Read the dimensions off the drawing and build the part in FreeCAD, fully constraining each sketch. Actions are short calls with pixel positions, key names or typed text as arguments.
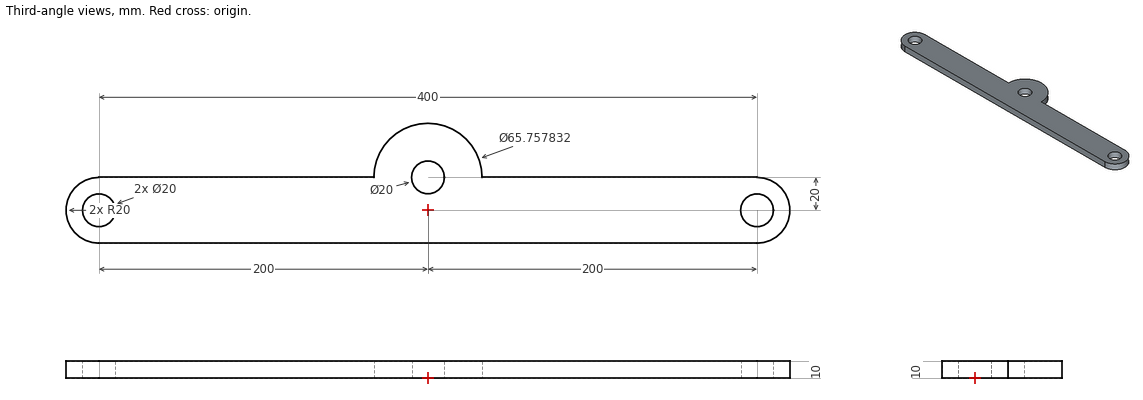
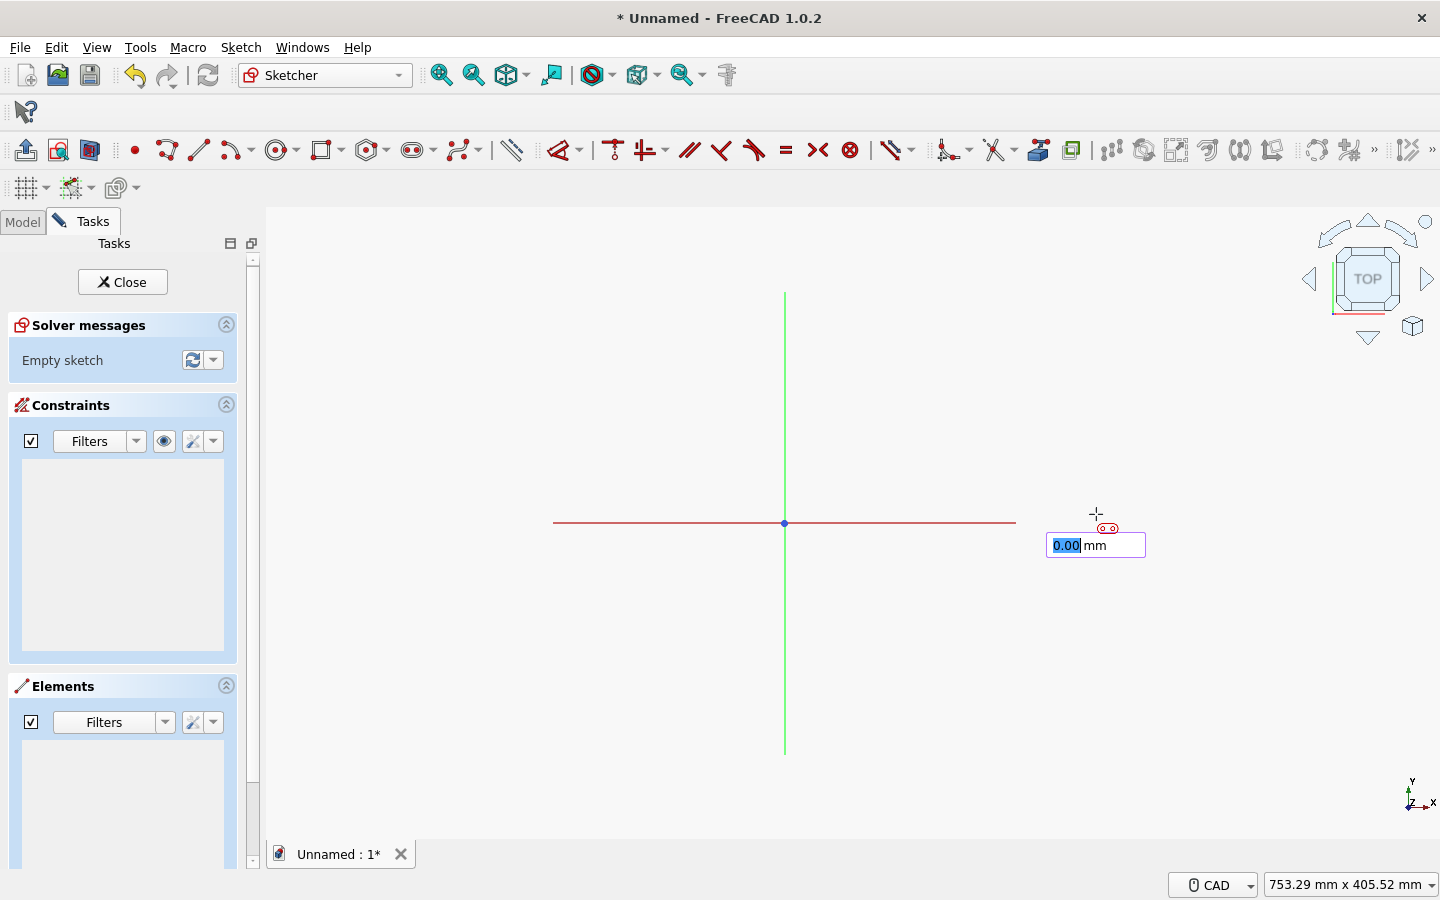
click(878, 492)
key(Escape)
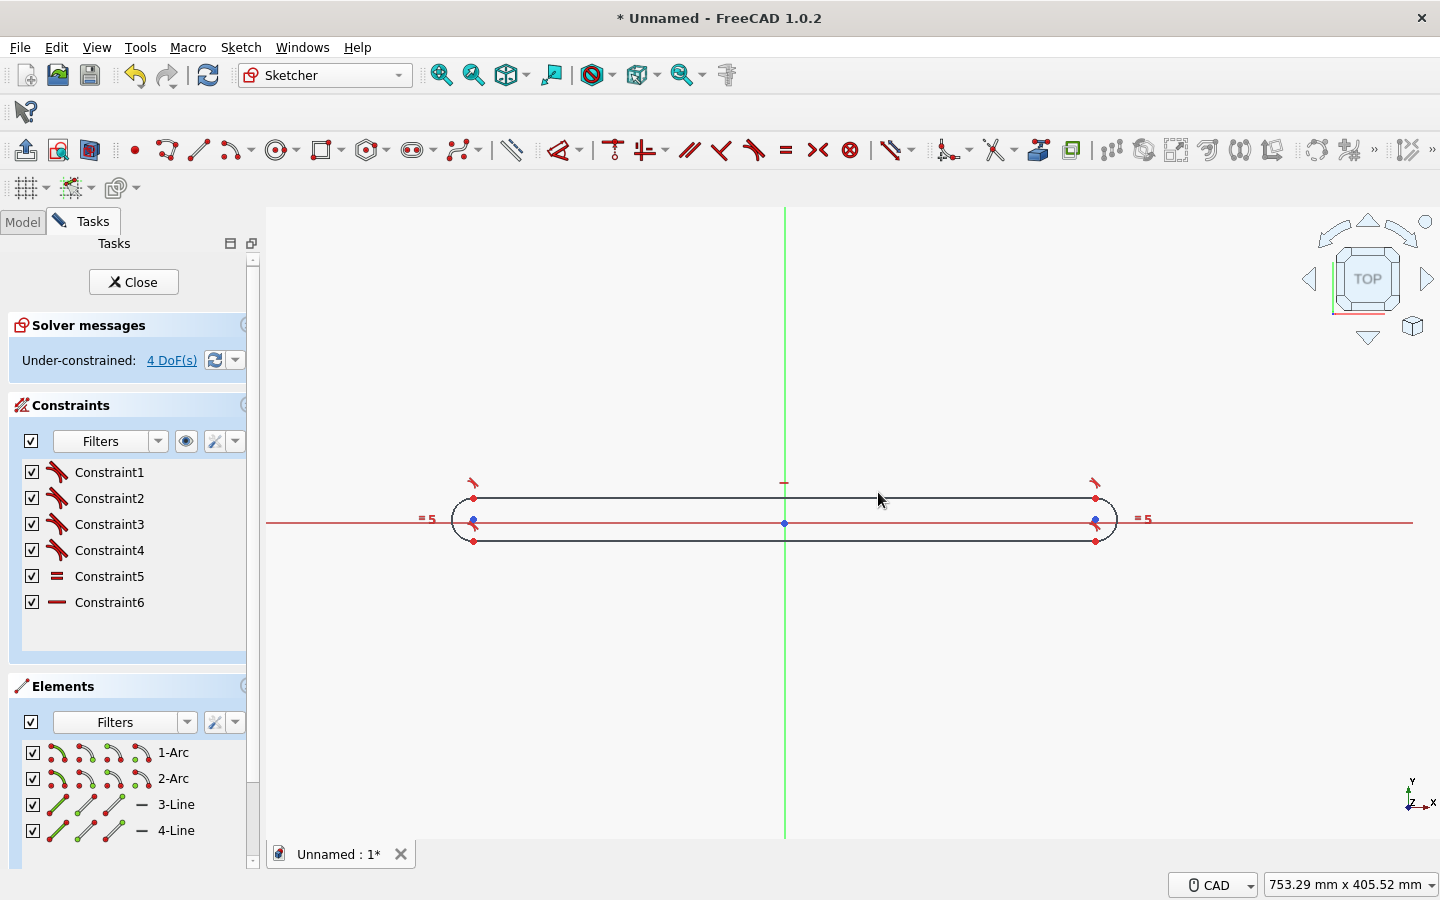
click(473, 520)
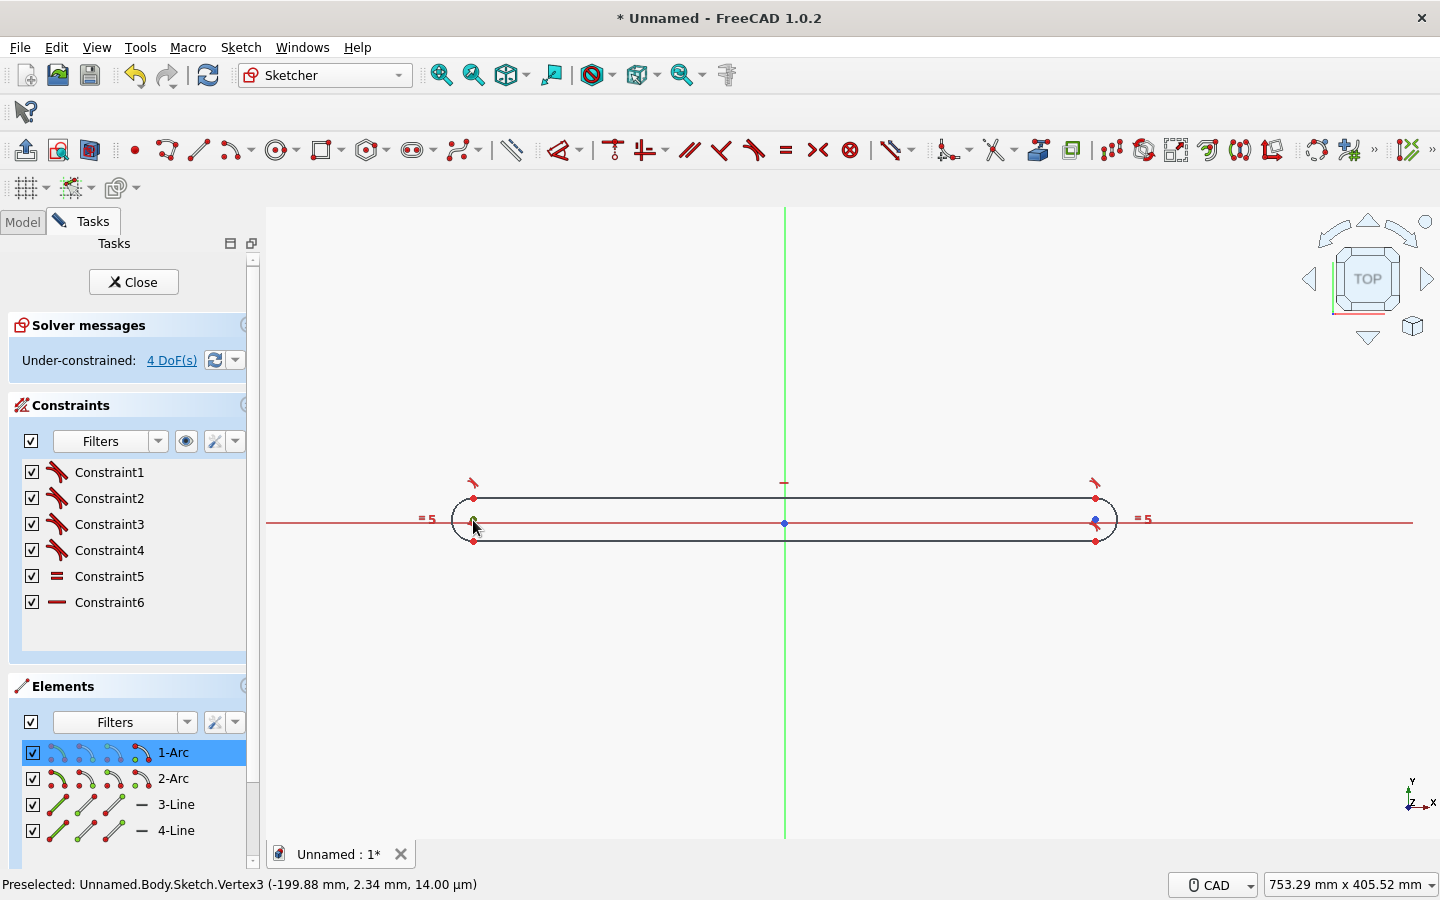
click(364, 523)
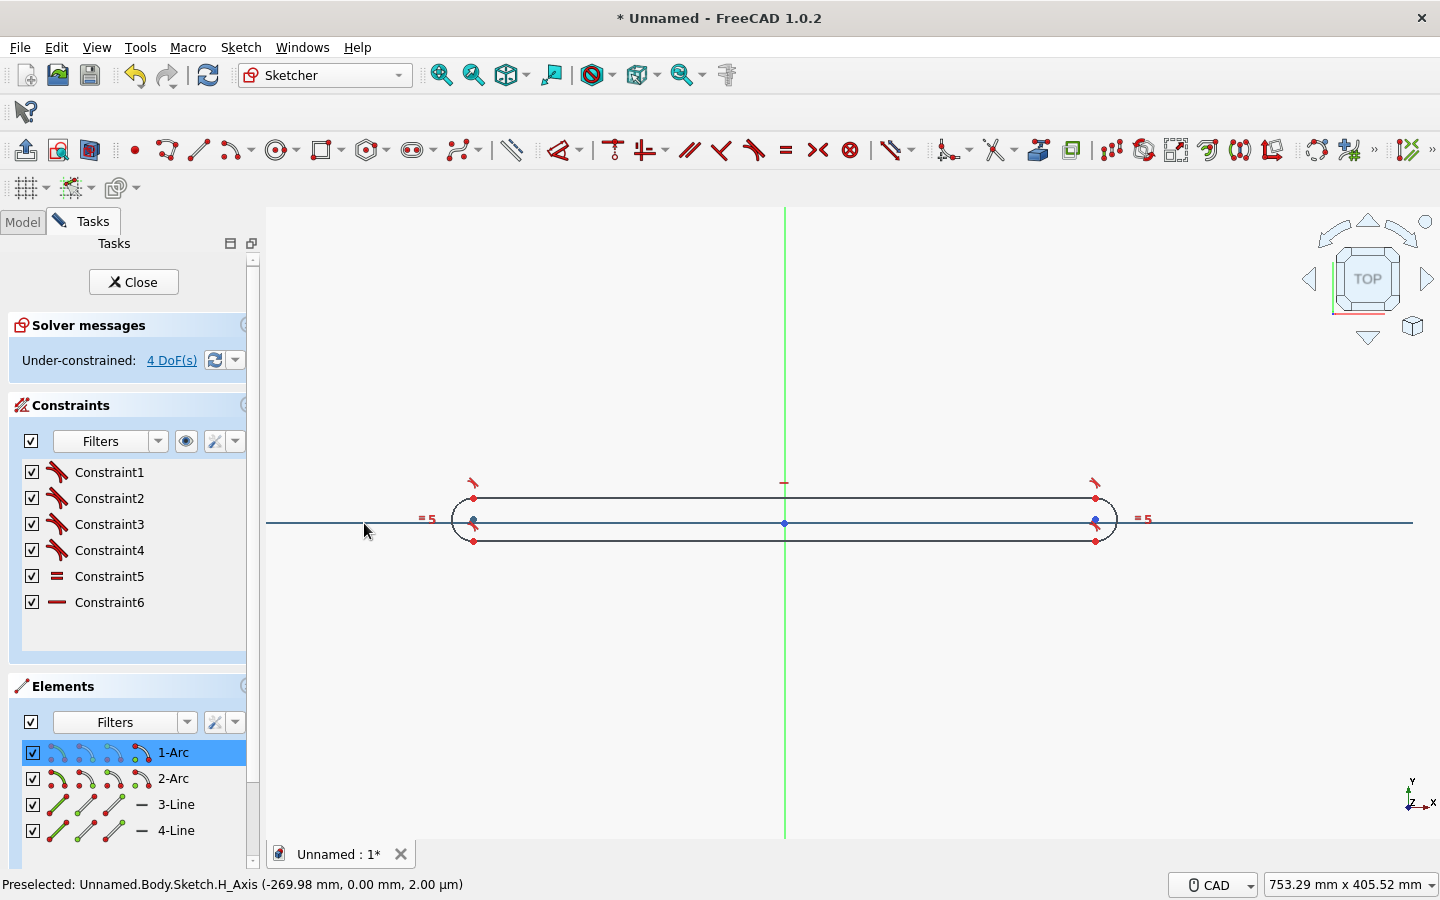
click(614, 150)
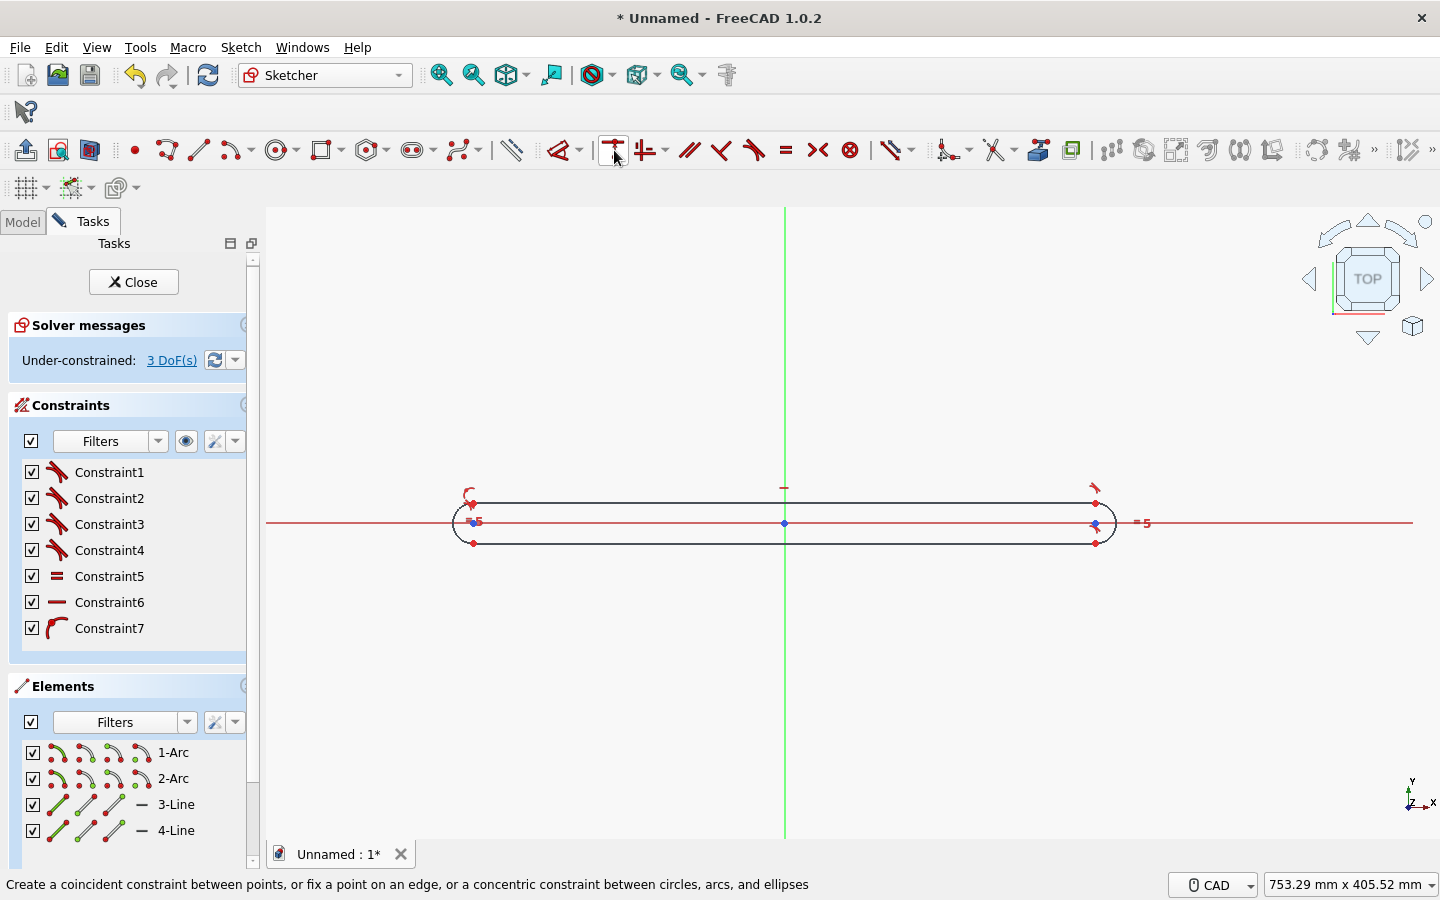
scroll(457, 511, up, 2)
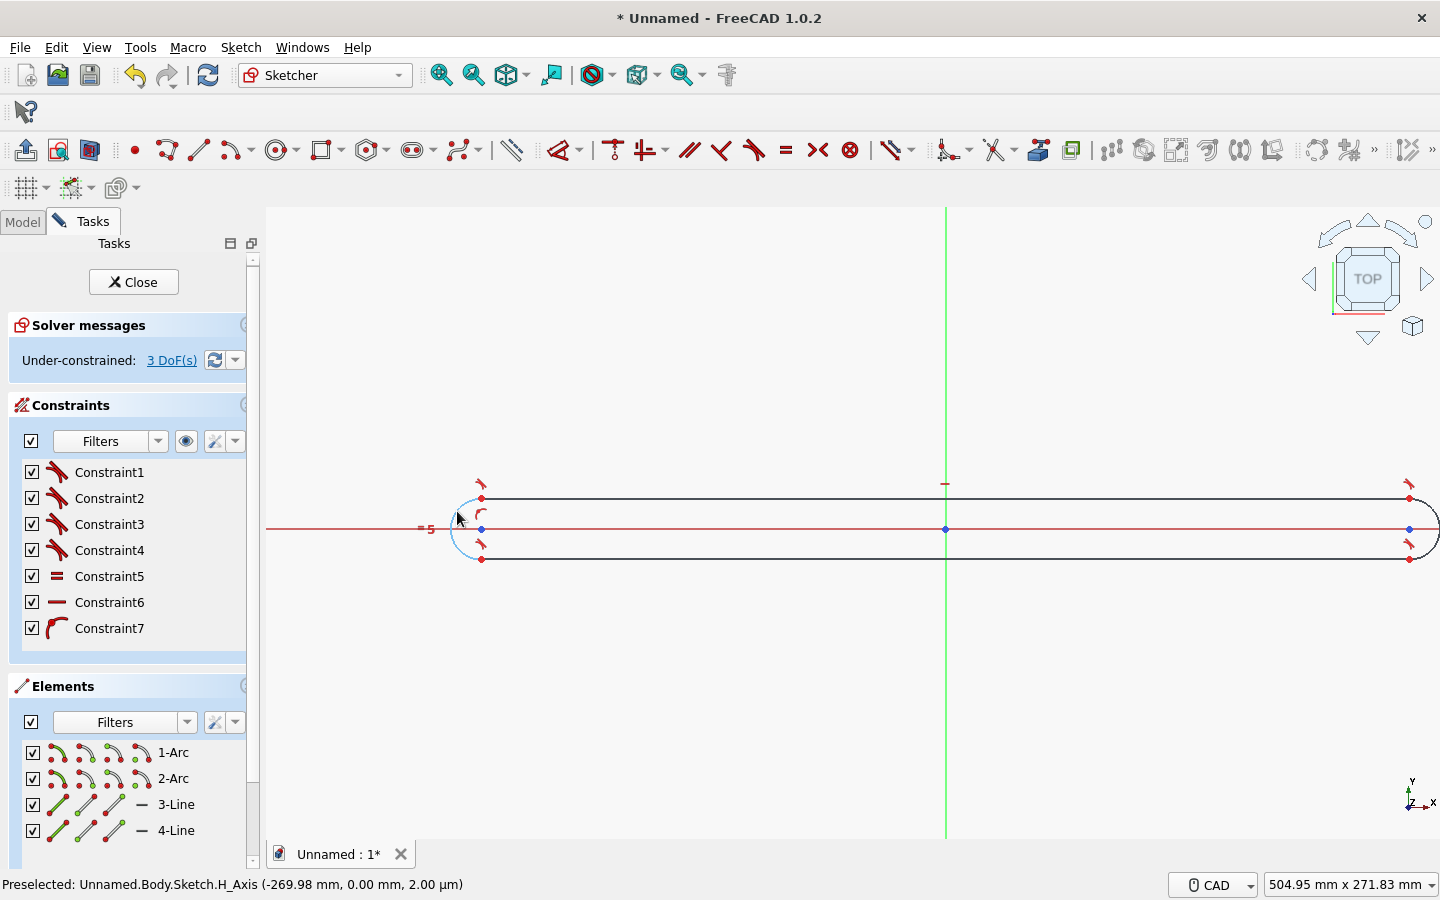
click(457, 511)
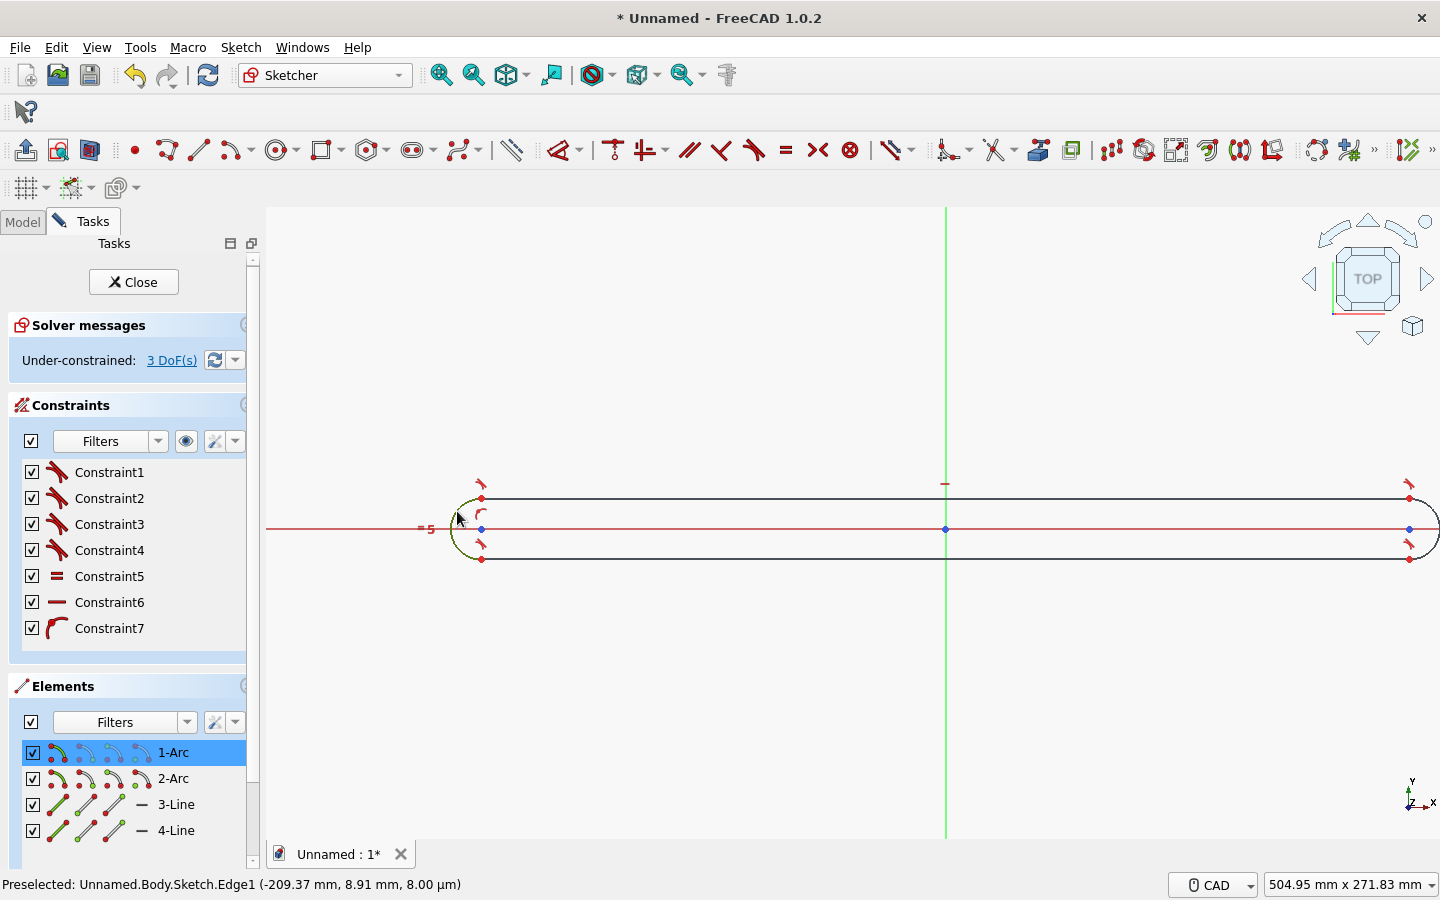
key(k)
key(r)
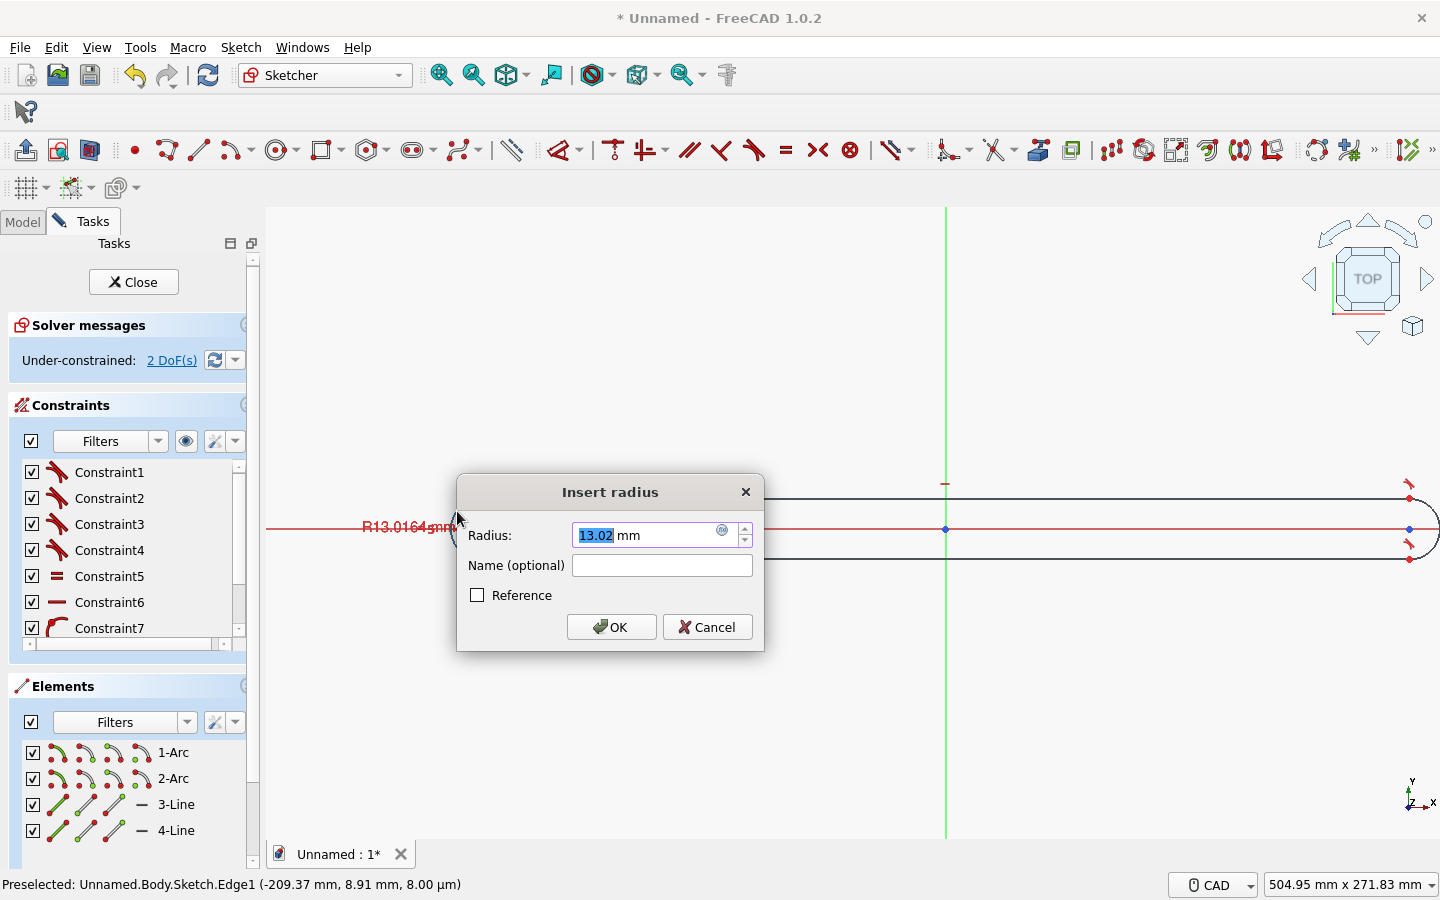
text(20)
key(Return)